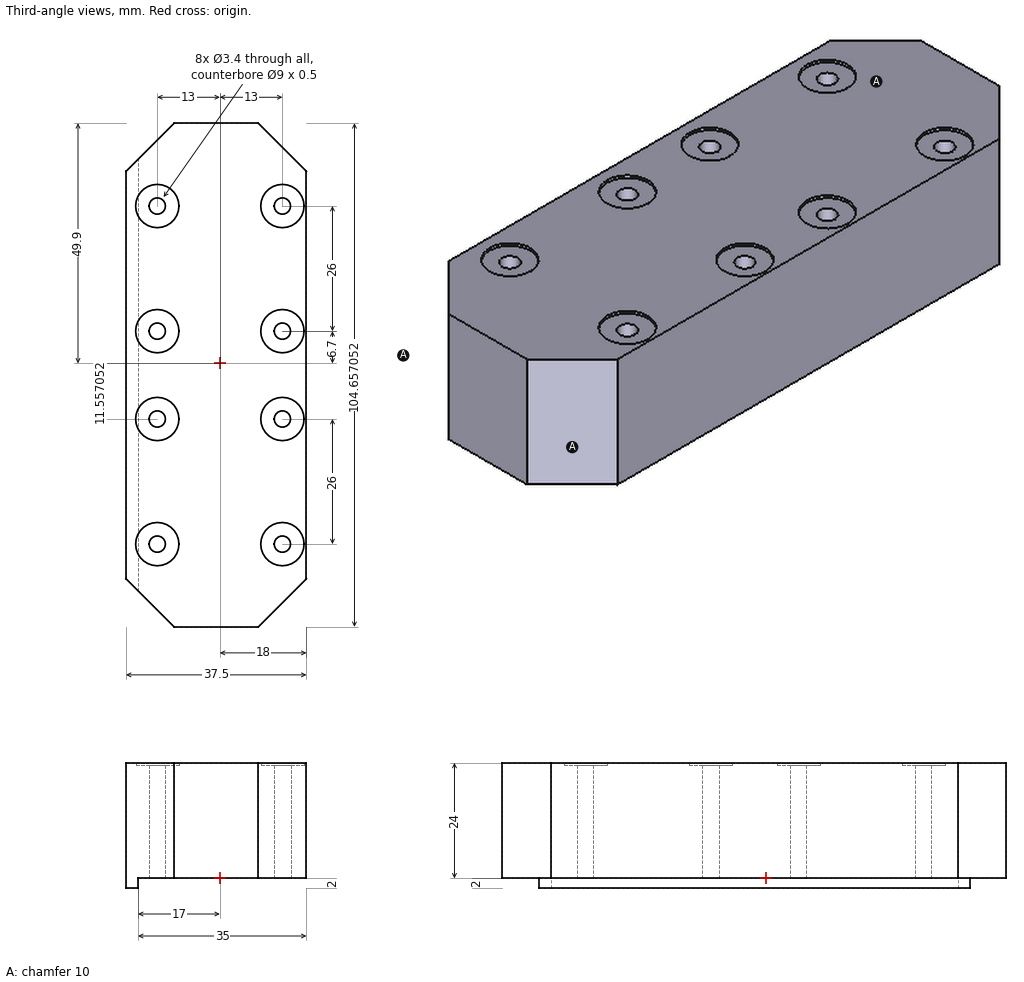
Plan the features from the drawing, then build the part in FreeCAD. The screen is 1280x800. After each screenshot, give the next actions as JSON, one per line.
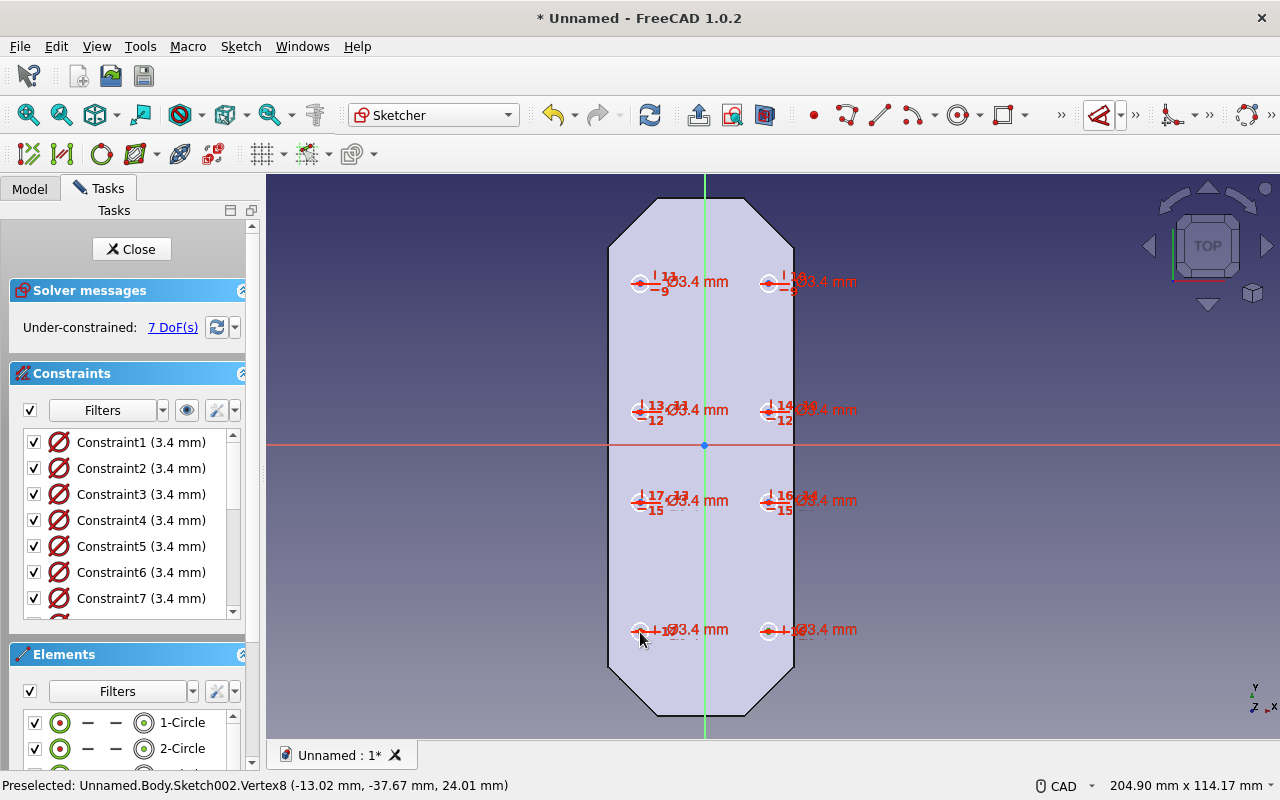
{"action": "key", "text": "h"}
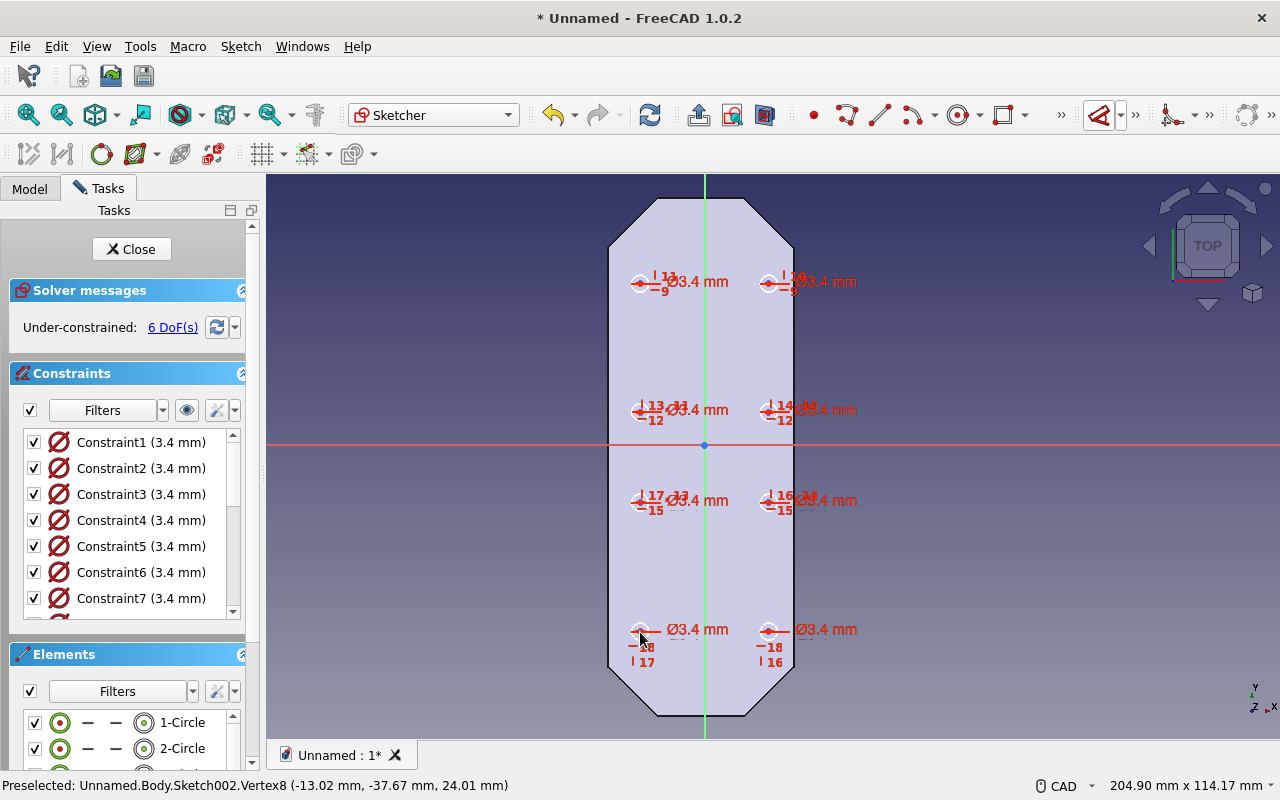
{"action": "left_click", "coordinate": [640, 284]}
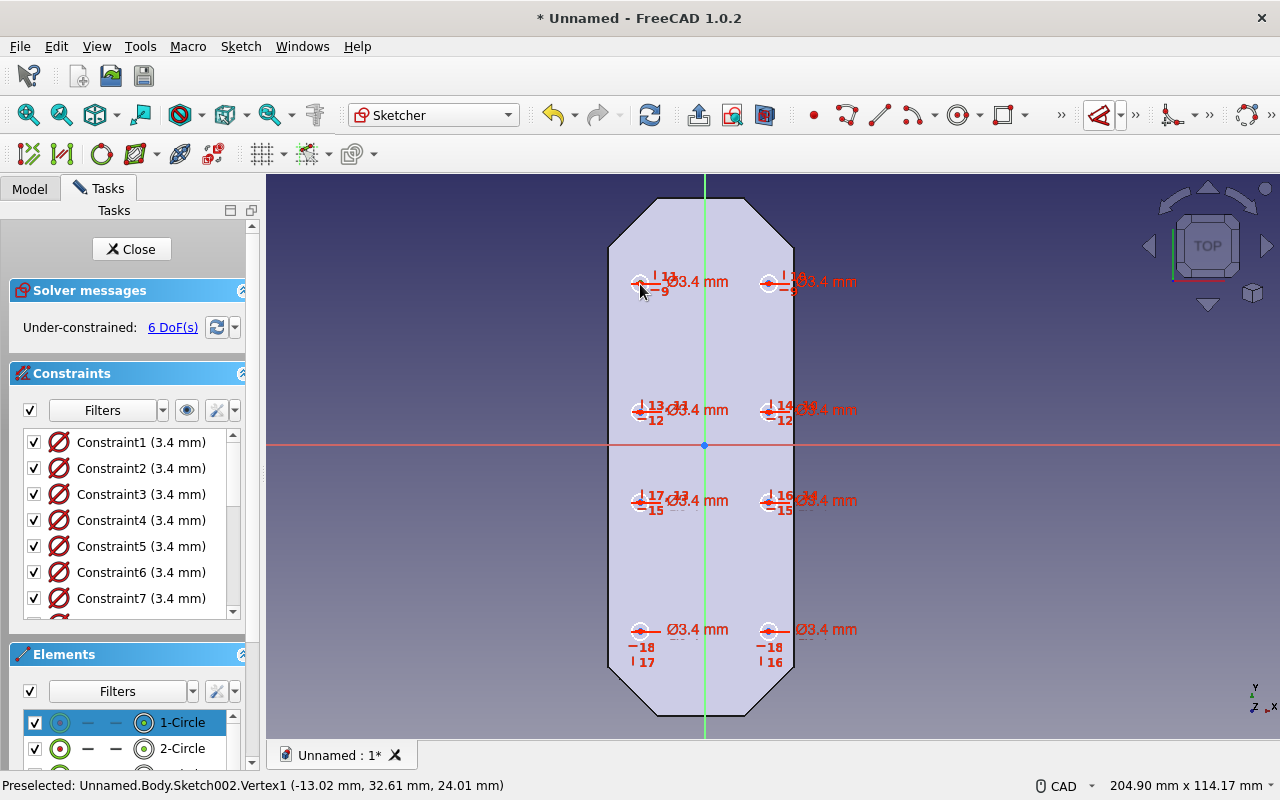
{"action": "left_click", "coordinate": [1120, 116]}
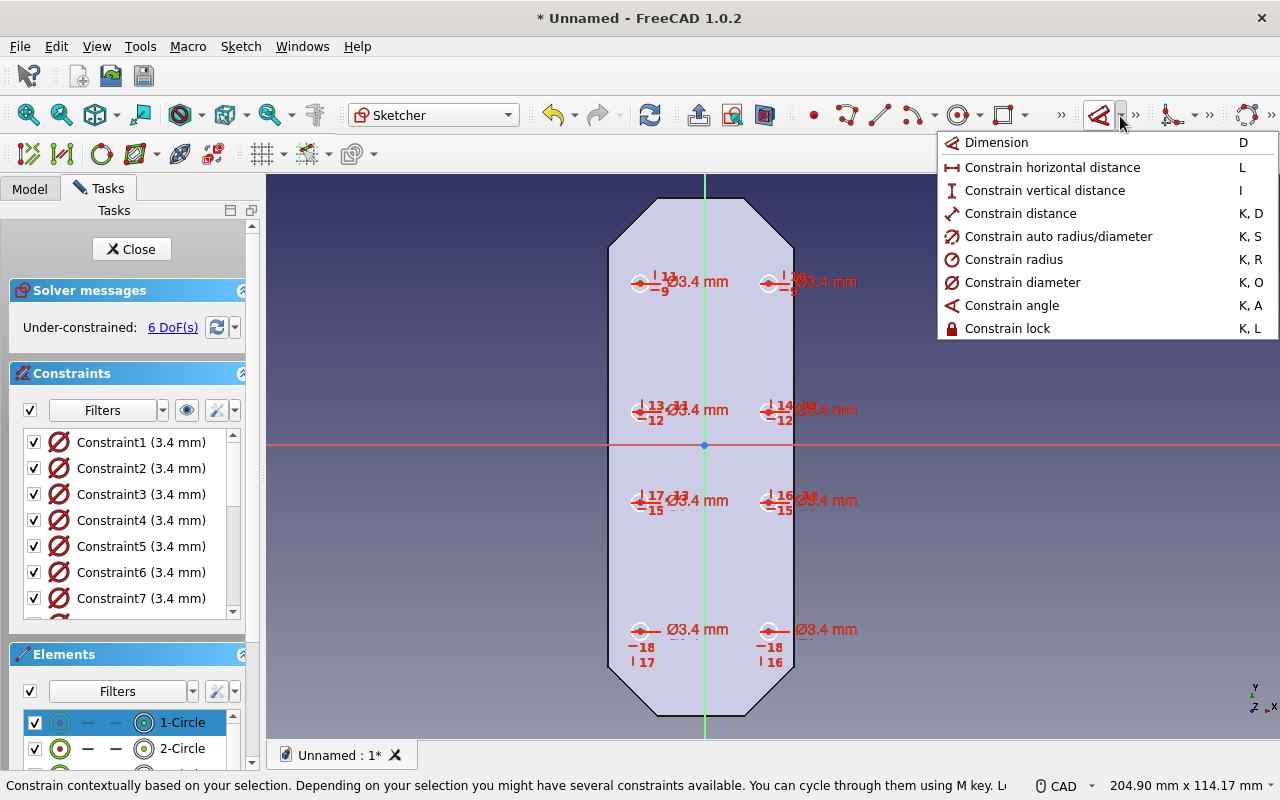
{"action": "left_click", "coordinate": [1108, 168]}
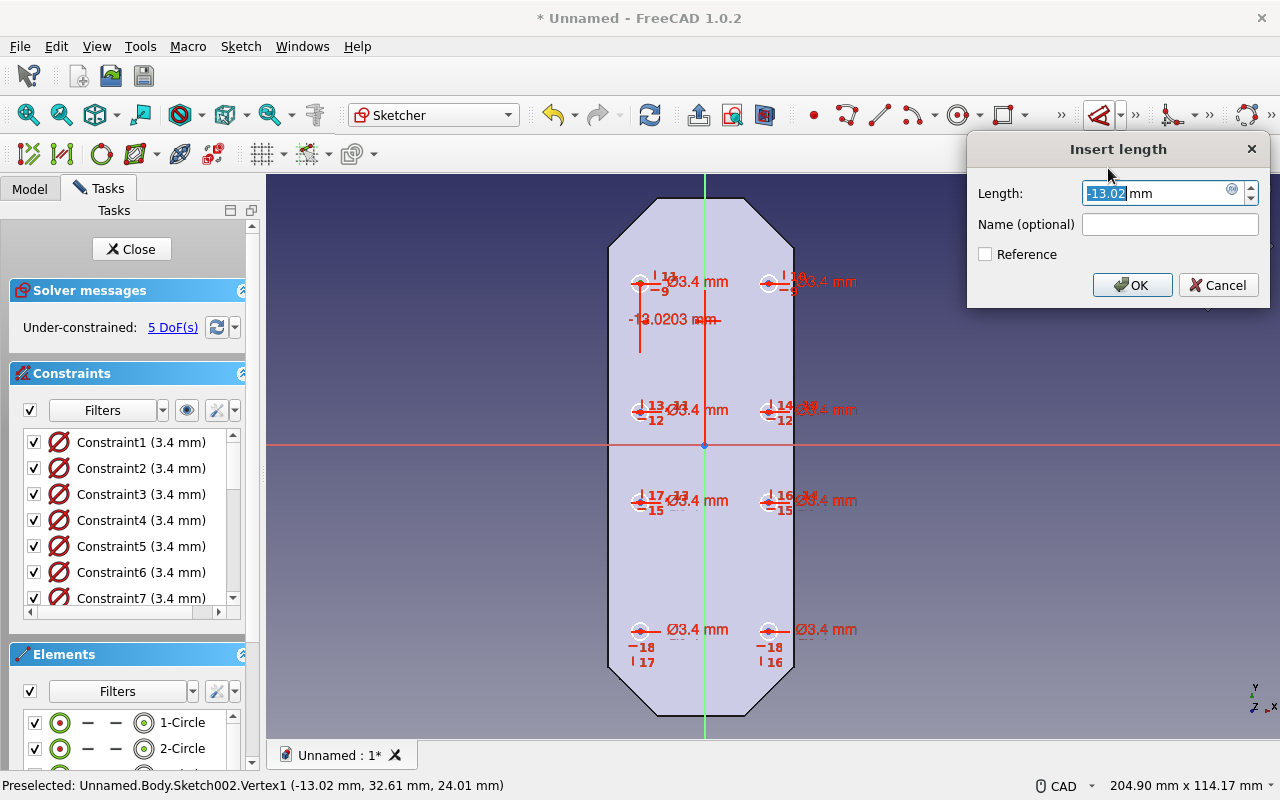
{"action": "type", "text": "-13"}
{"action": "key", "text": "Return"}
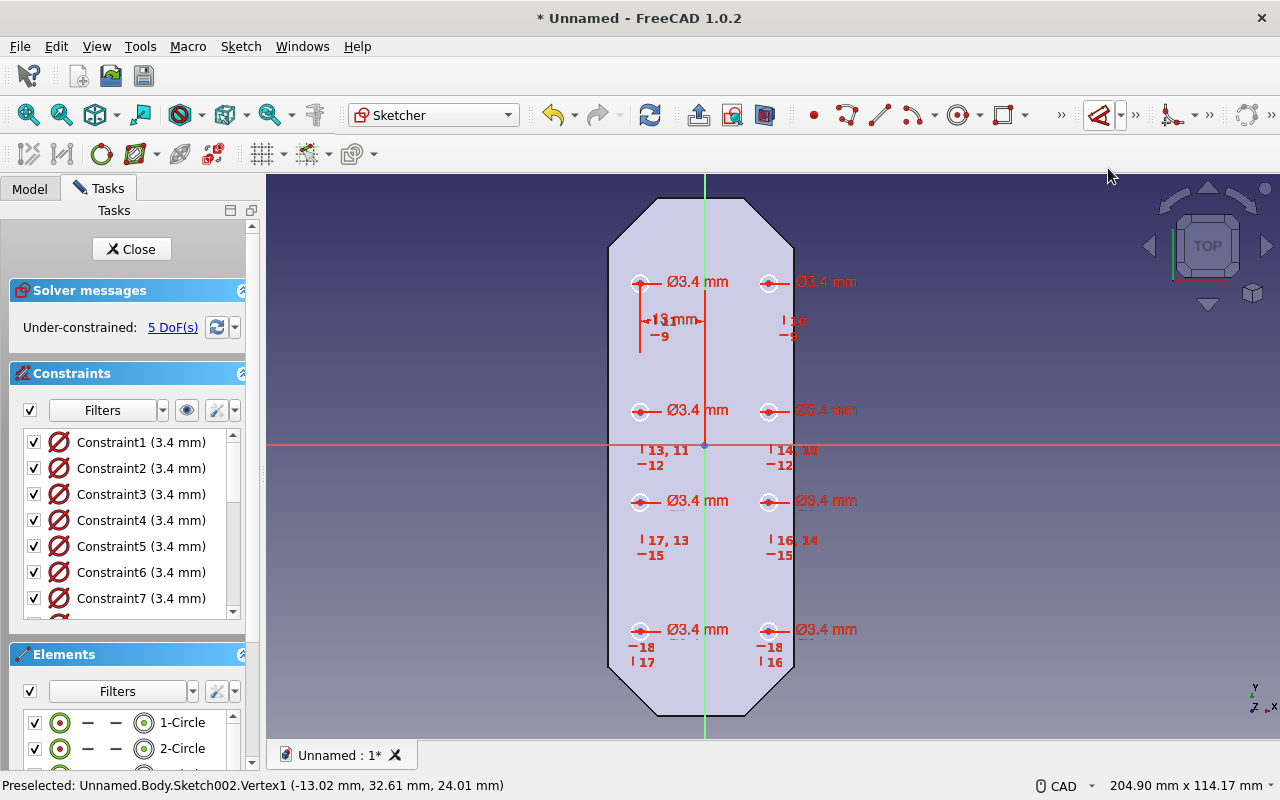
{"action": "left_click", "coordinate": [769, 284]}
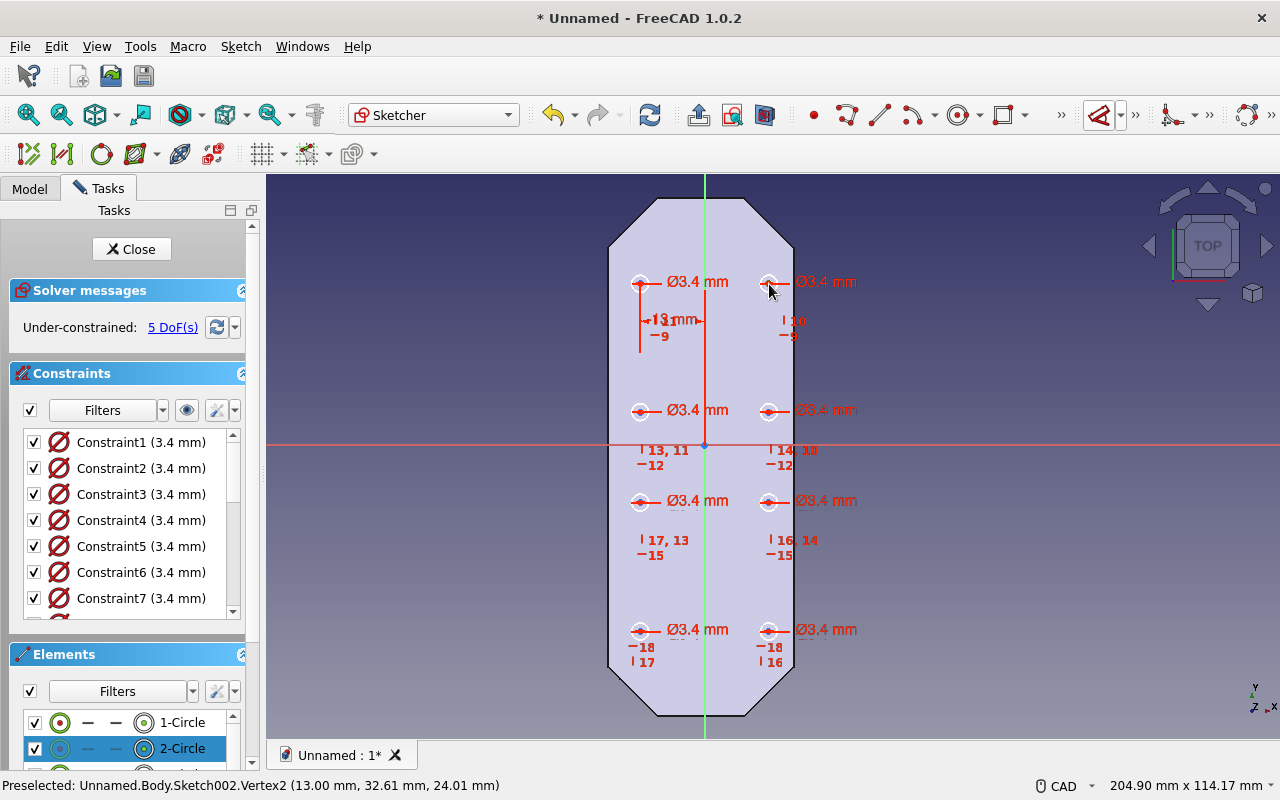
{"action": "left_click", "coordinate": [1120, 116]}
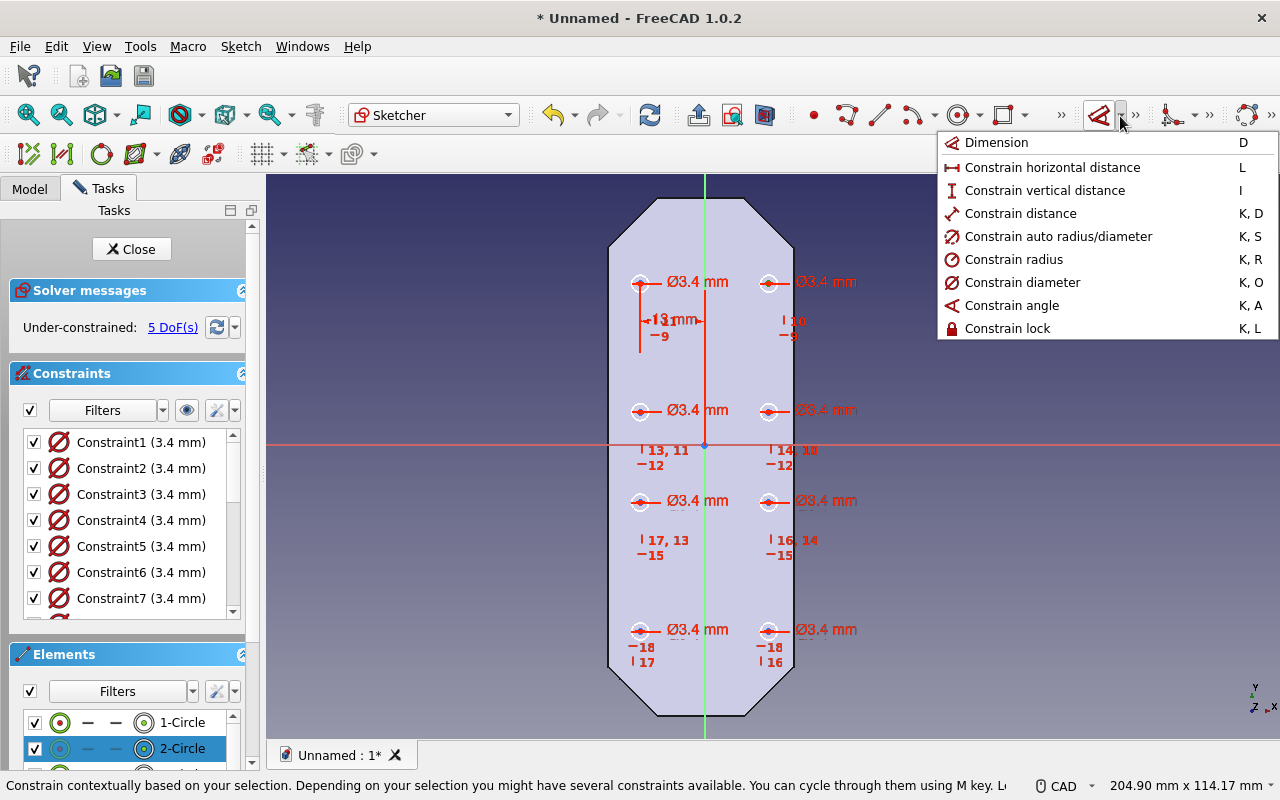
{"action": "left_click", "coordinate": [1108, 168]}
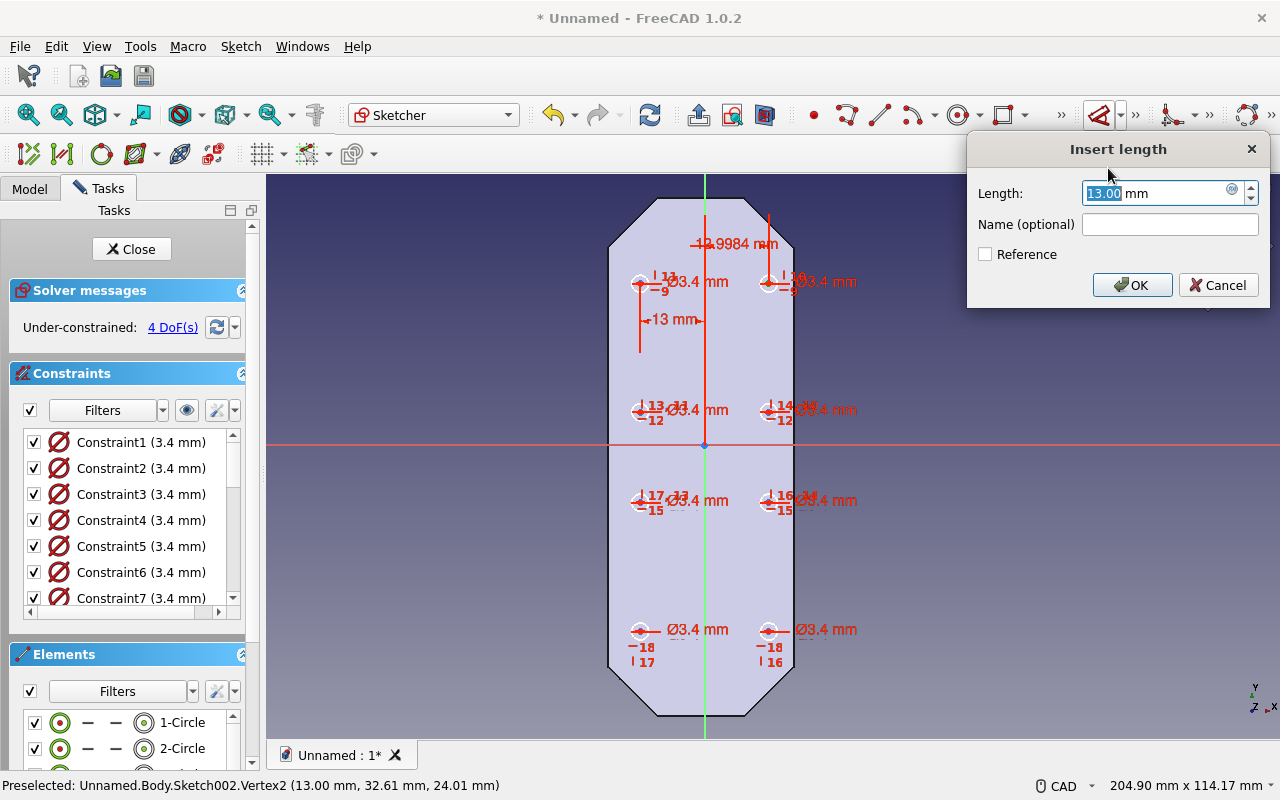
{"action": "type", "text": "13"}
{"action": "key", "text": "Return"}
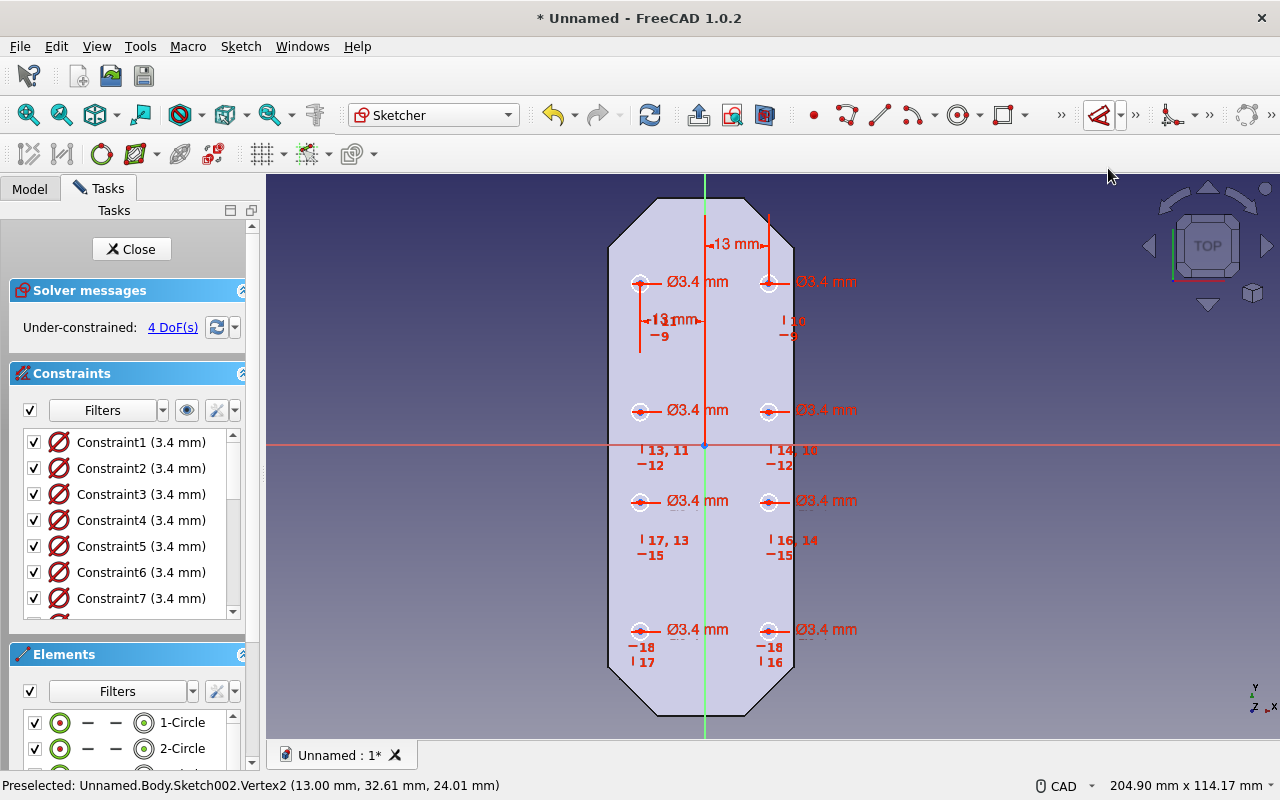
{"action": "left_click", "coordinate": [769, 412]}